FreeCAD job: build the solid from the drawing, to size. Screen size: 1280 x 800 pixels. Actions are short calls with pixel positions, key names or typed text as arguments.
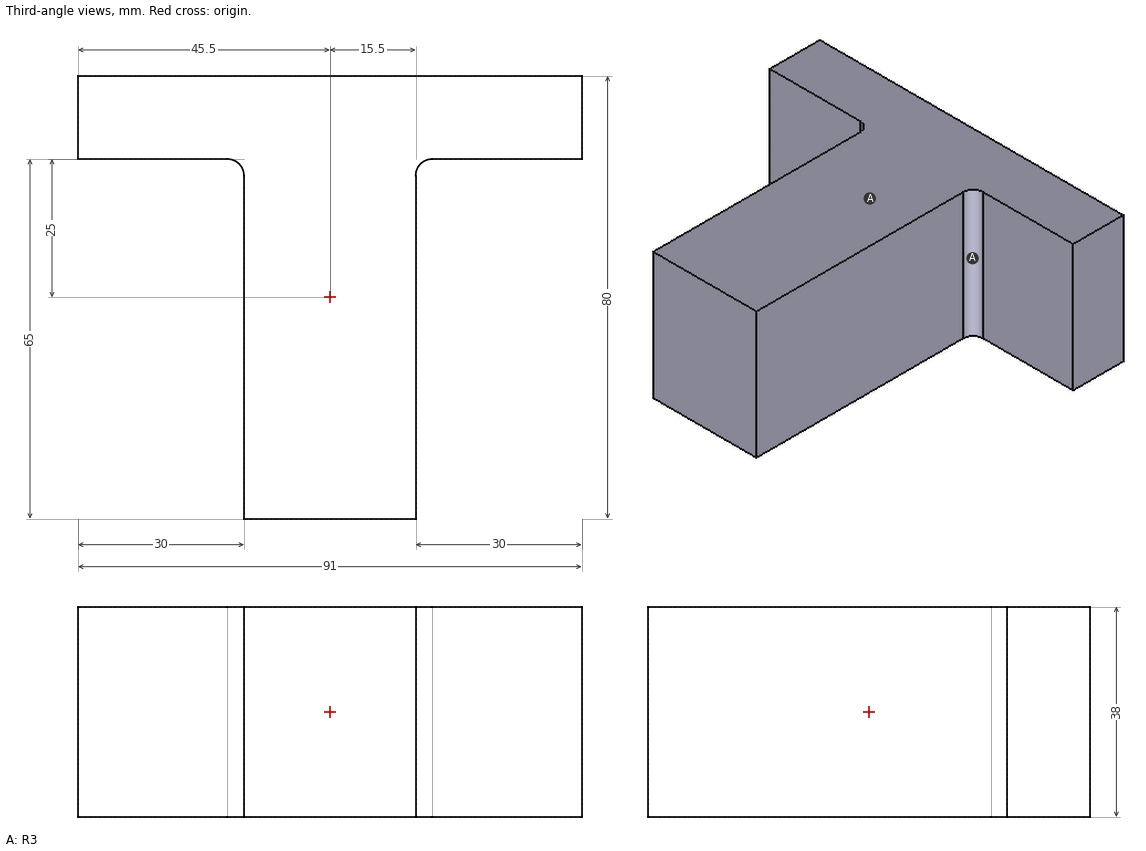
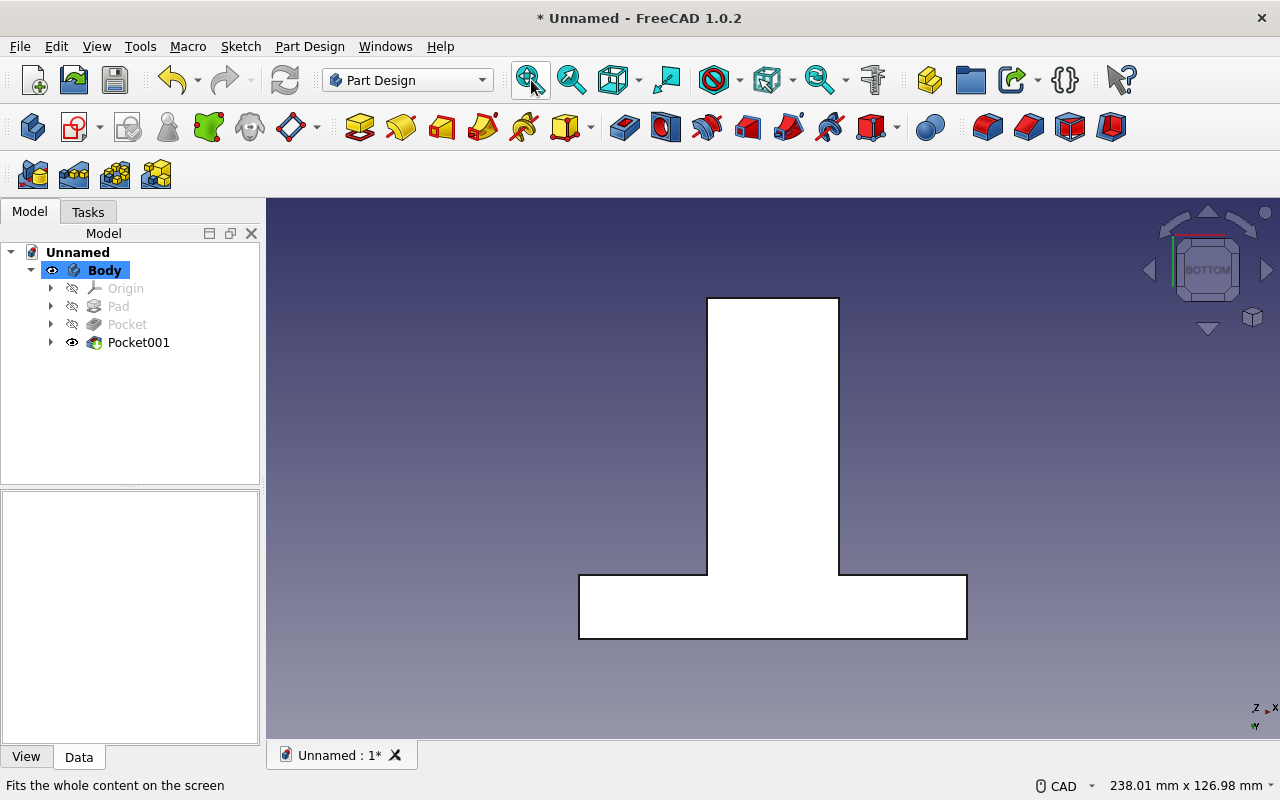
key(4)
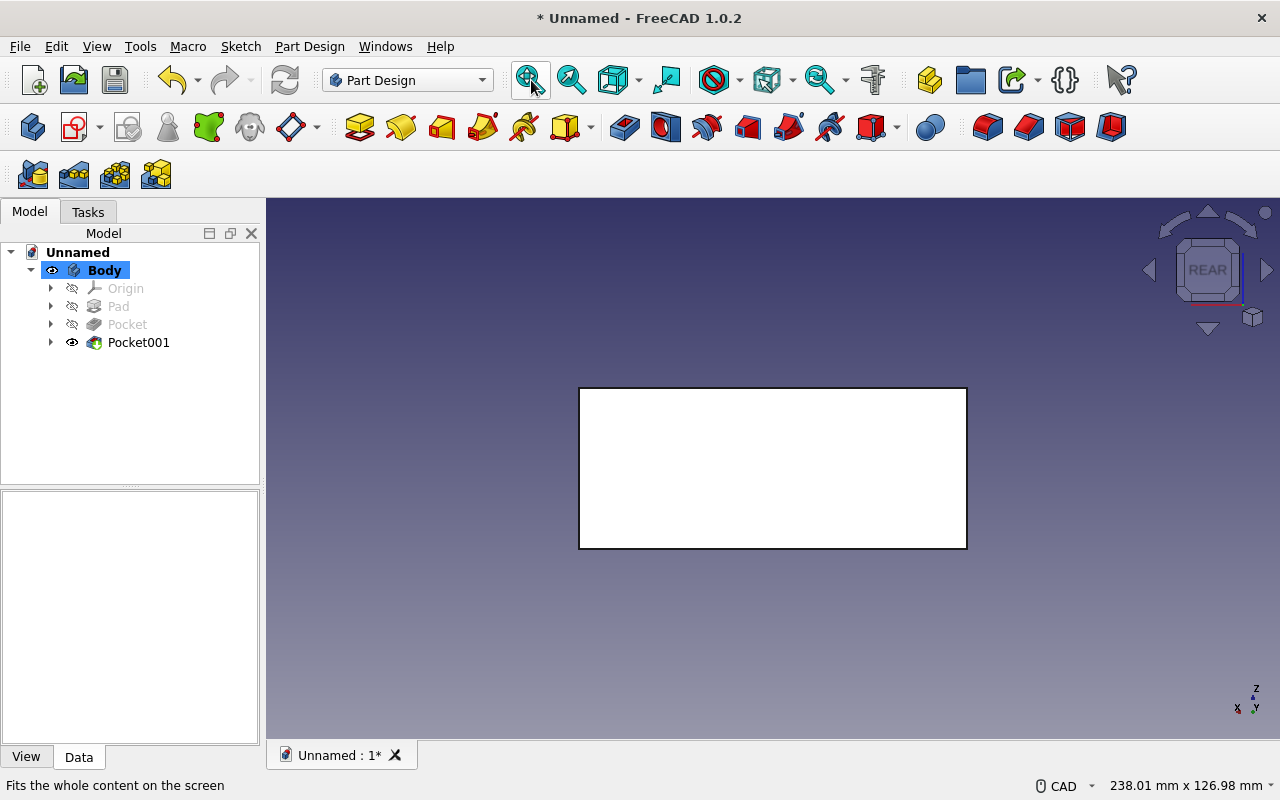
click(531, 80)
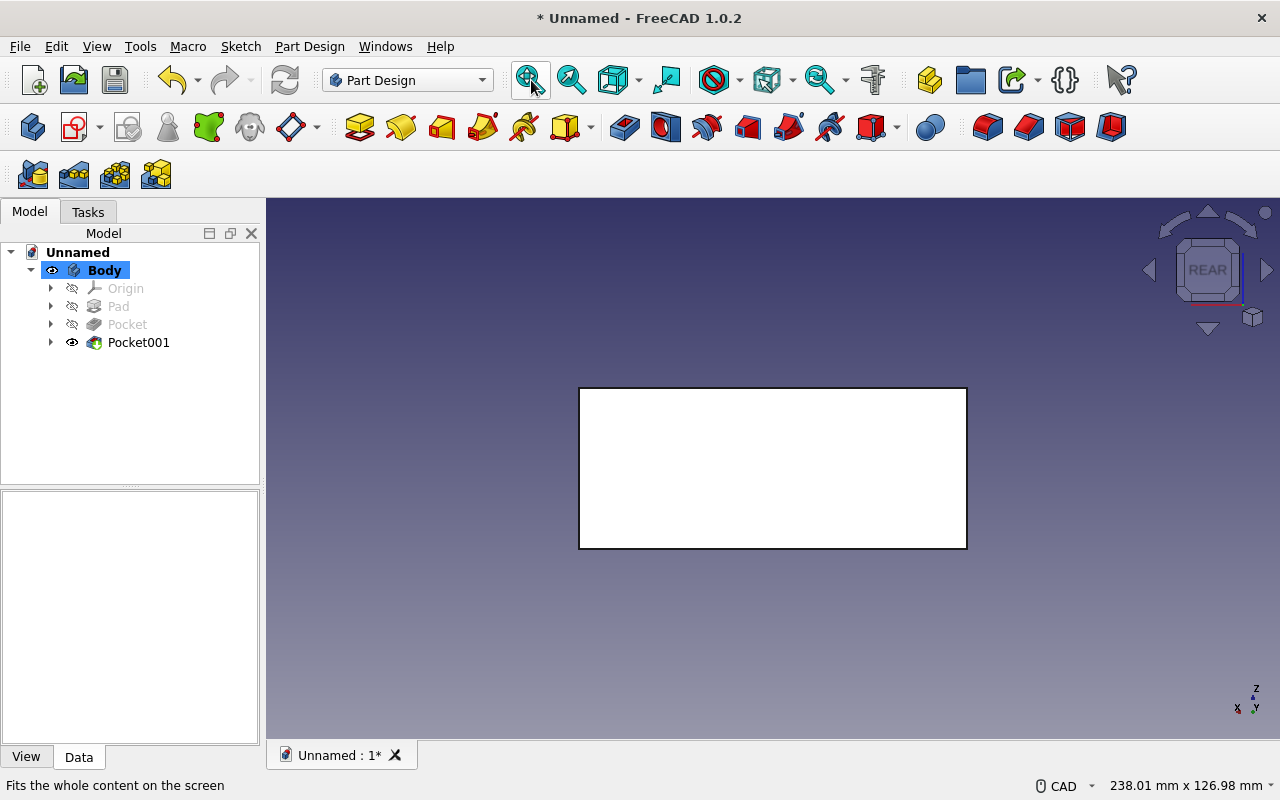
key(6)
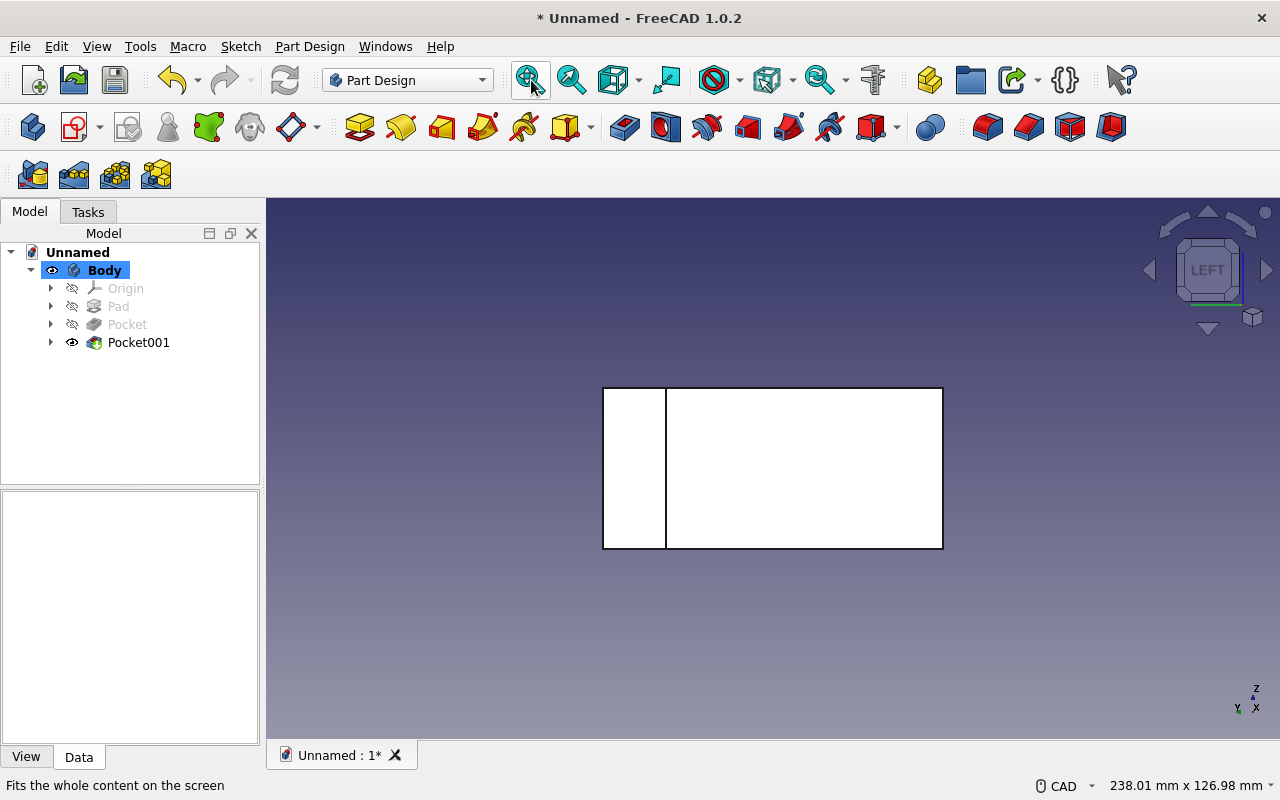
key(v)
key(f)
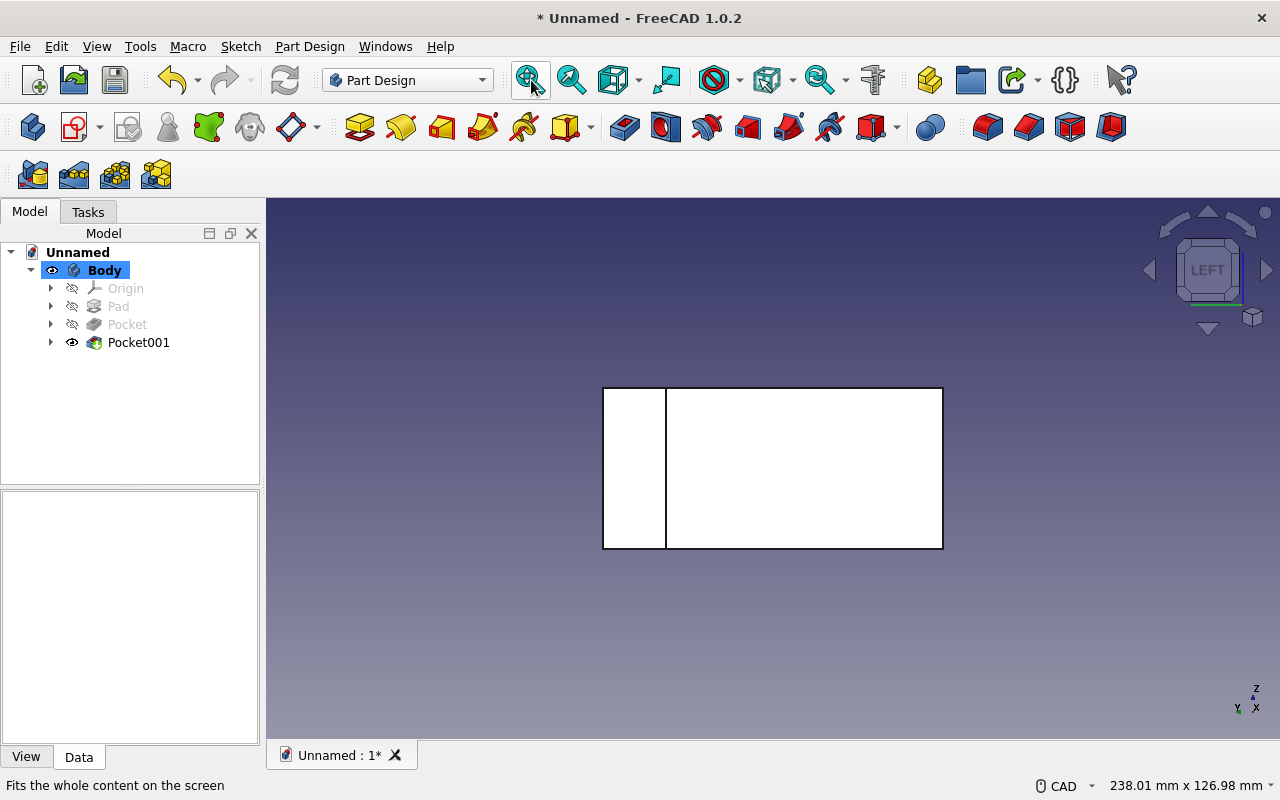
key(v)
key(3)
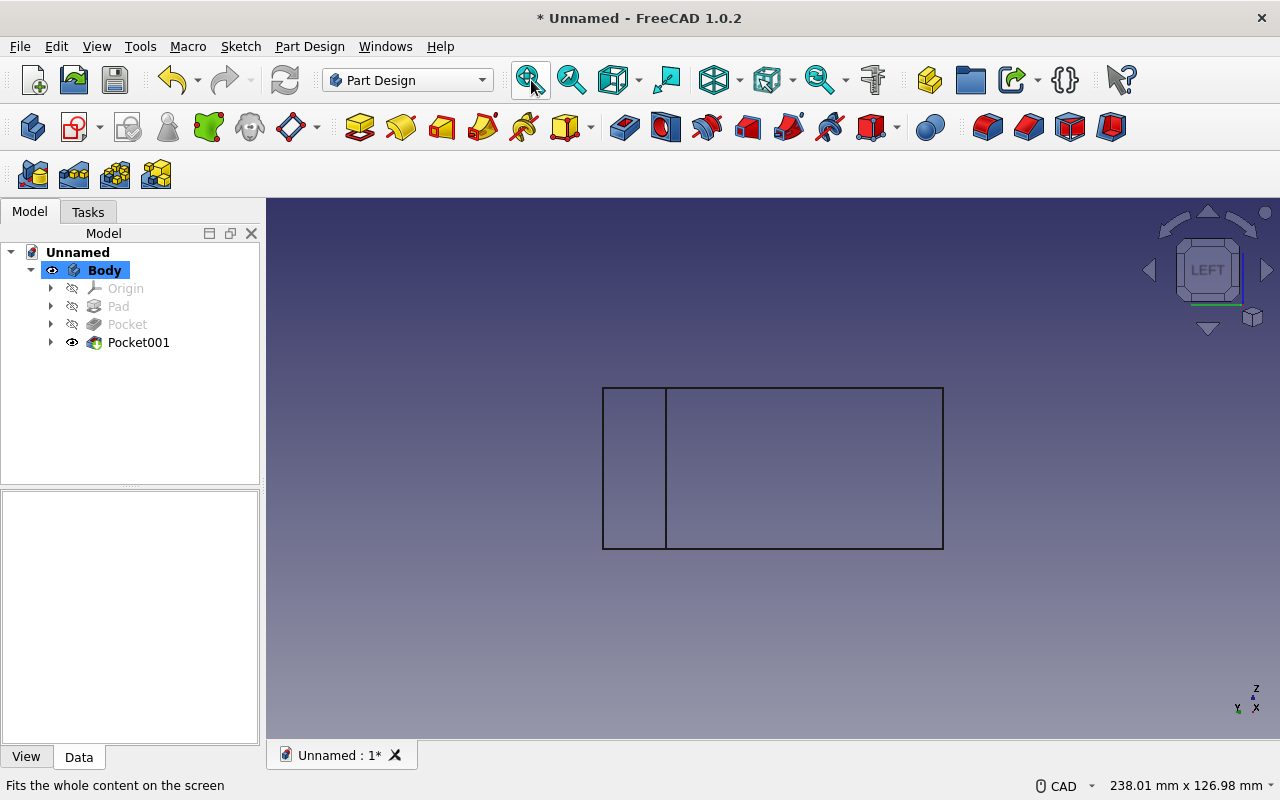
key(0)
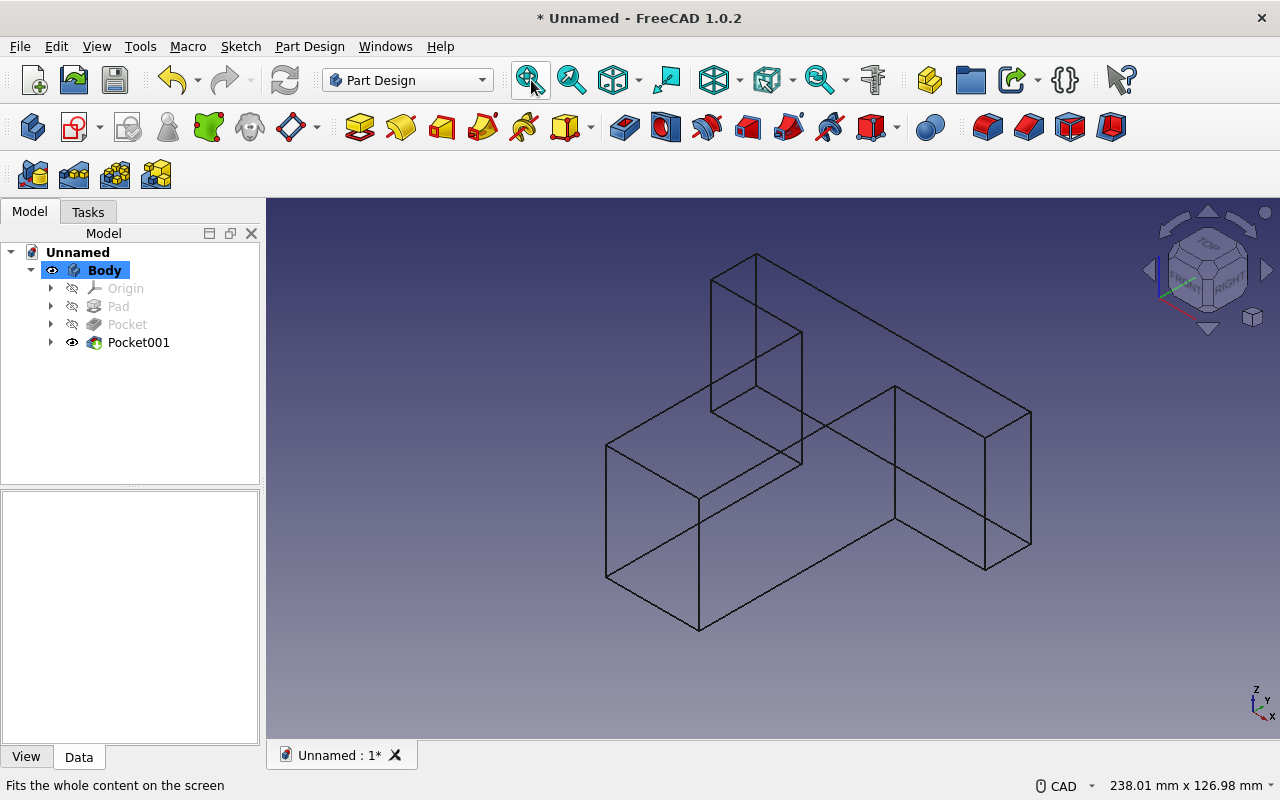
click(802, 397)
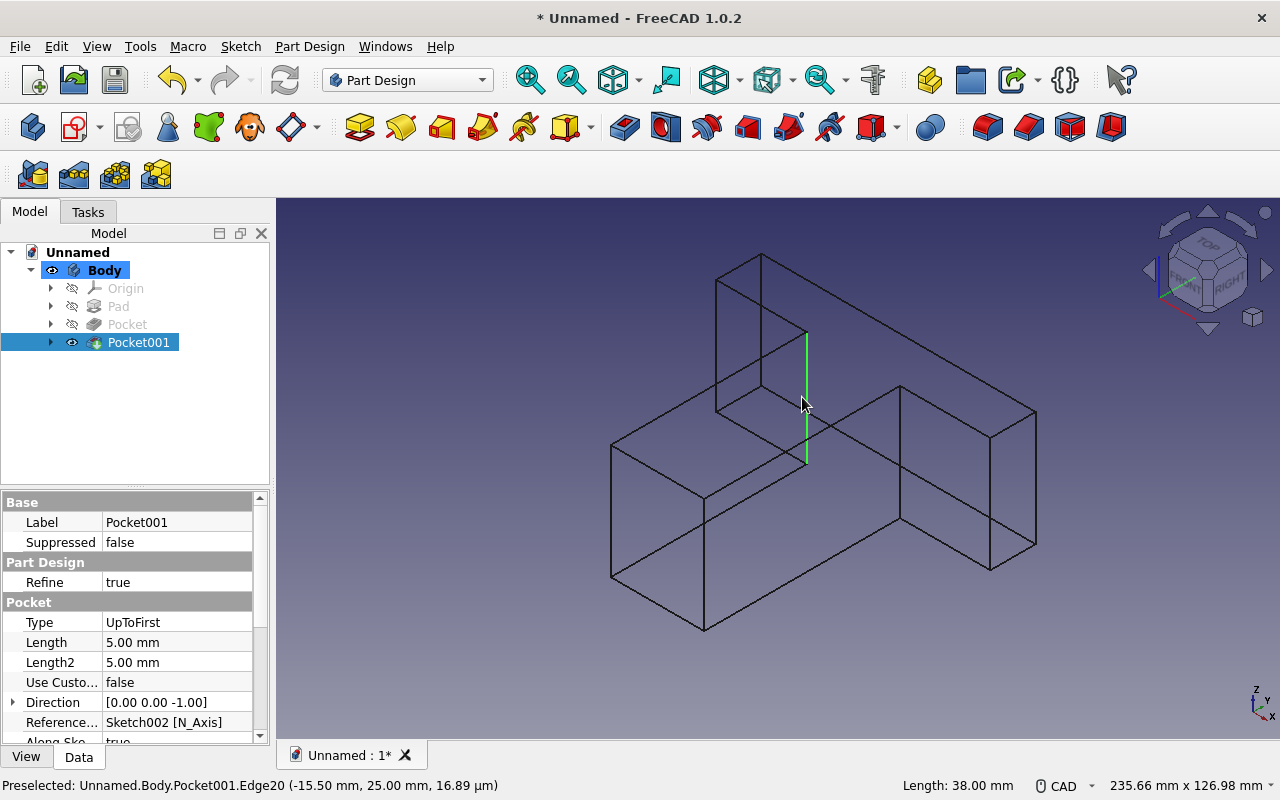
click(900, 451, ctrl)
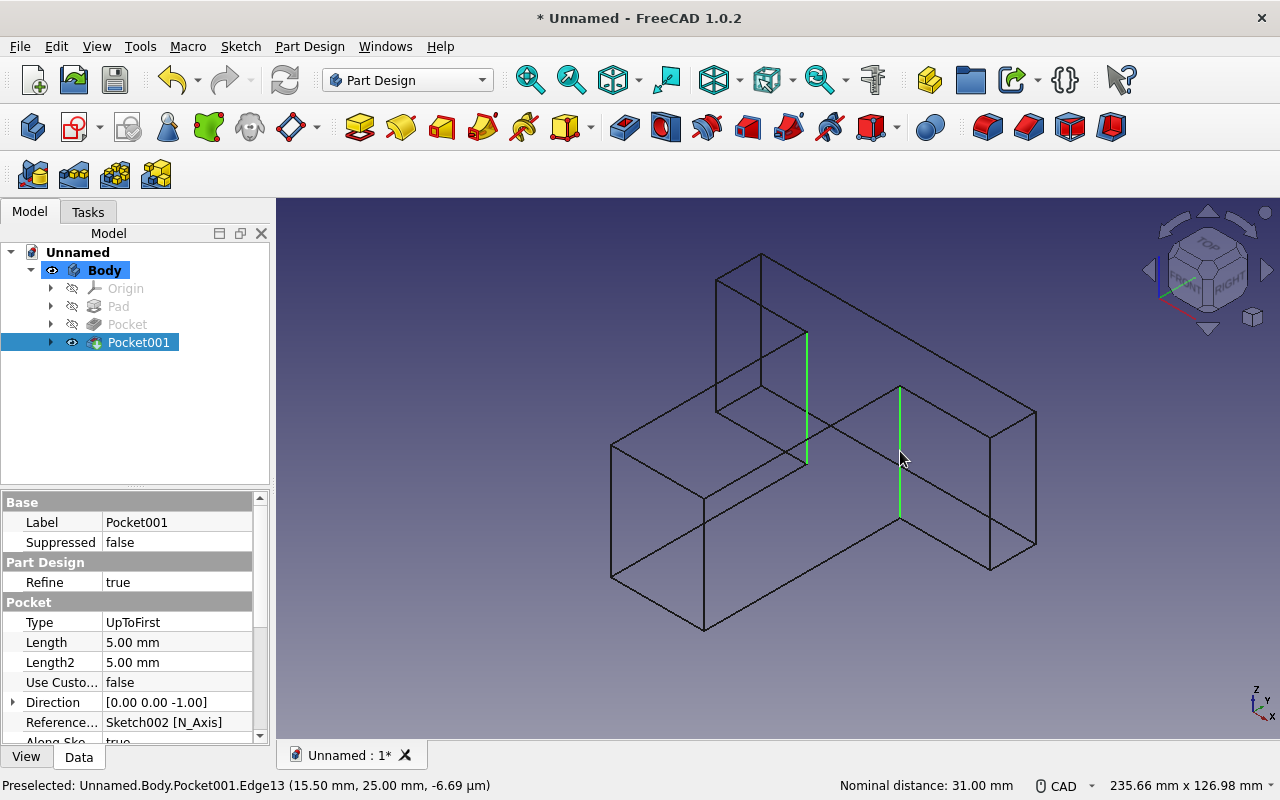
key(v)
key(1)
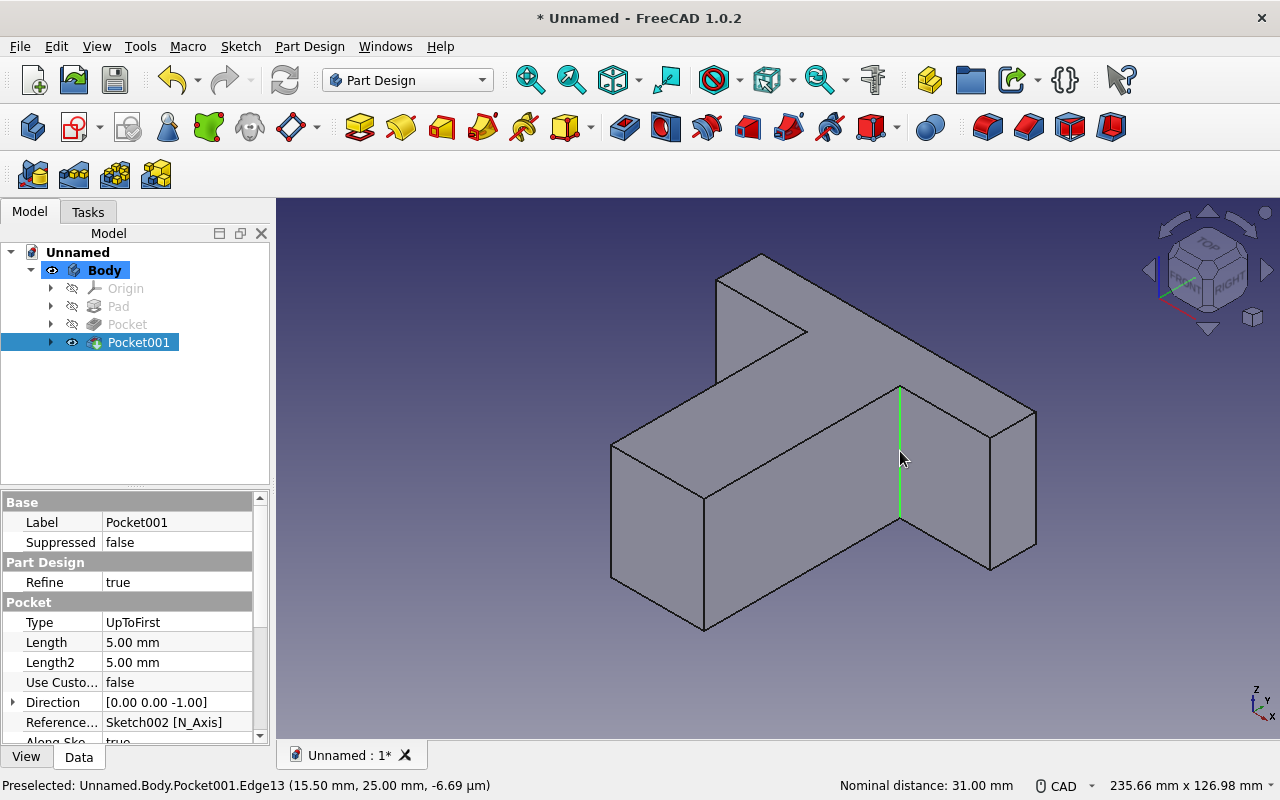
click(988, 128)